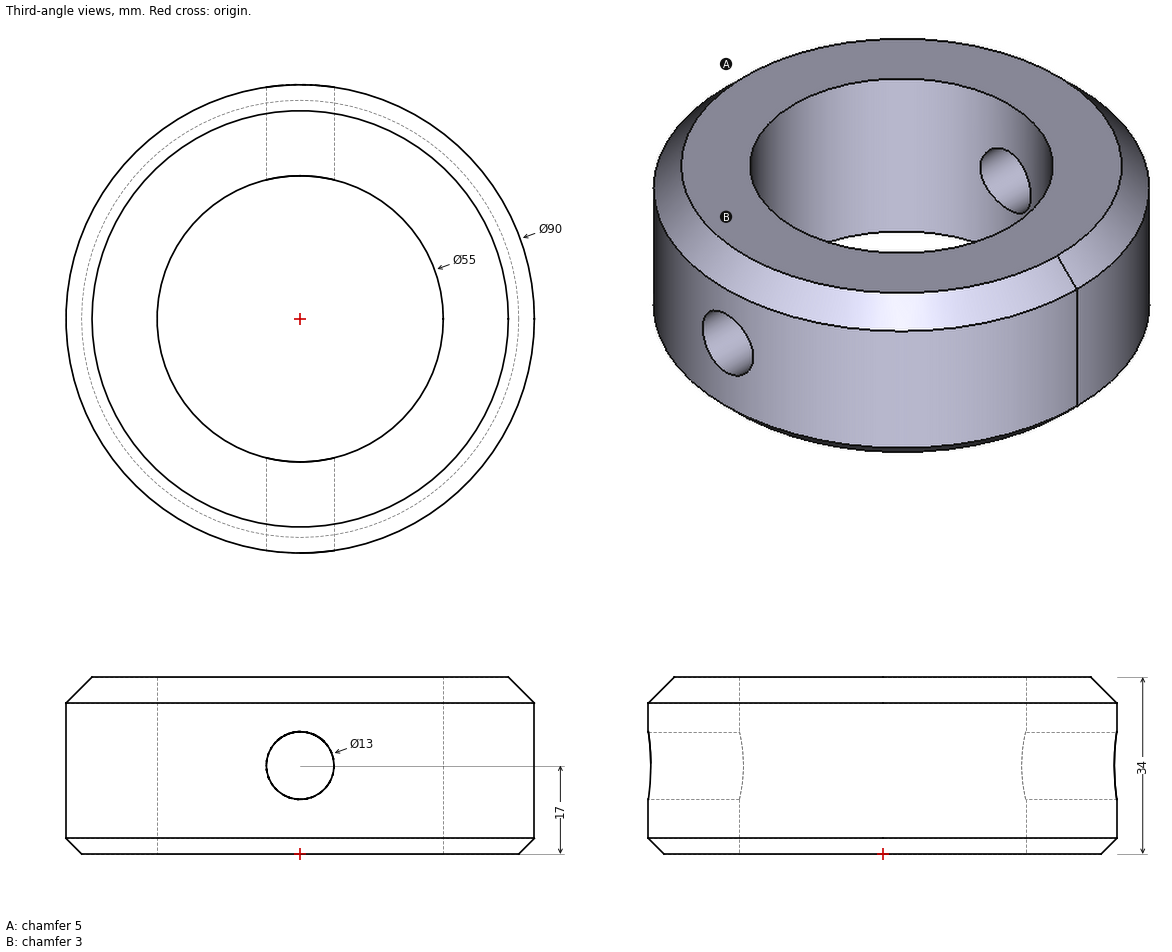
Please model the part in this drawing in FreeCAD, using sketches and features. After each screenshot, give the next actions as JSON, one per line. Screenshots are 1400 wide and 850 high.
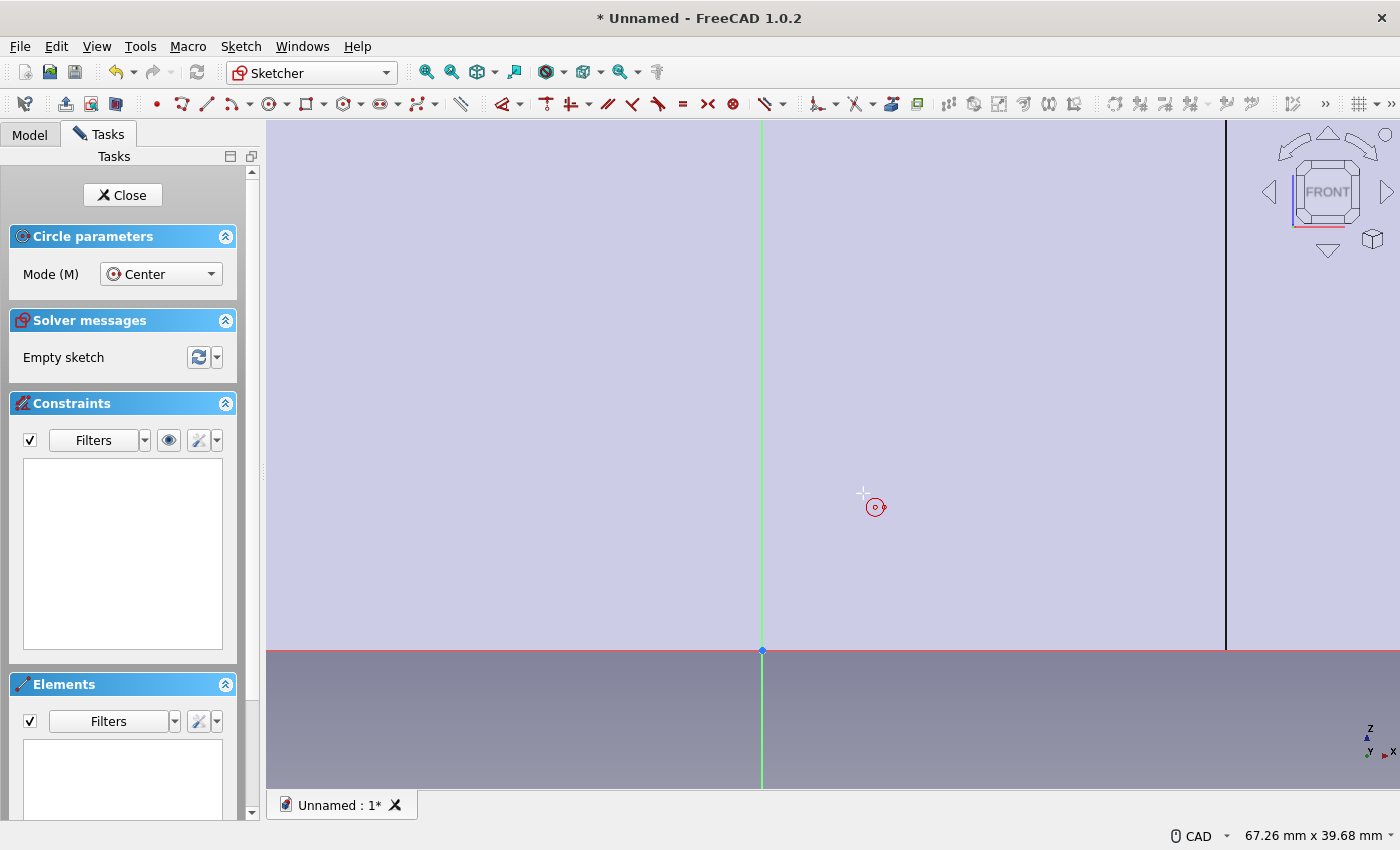
{"action": "left_click", "coordinate": [762, 364]}
{"action": "left_click", "coordinate": [840, 286]}
{"action": "key", "text": "Escape"}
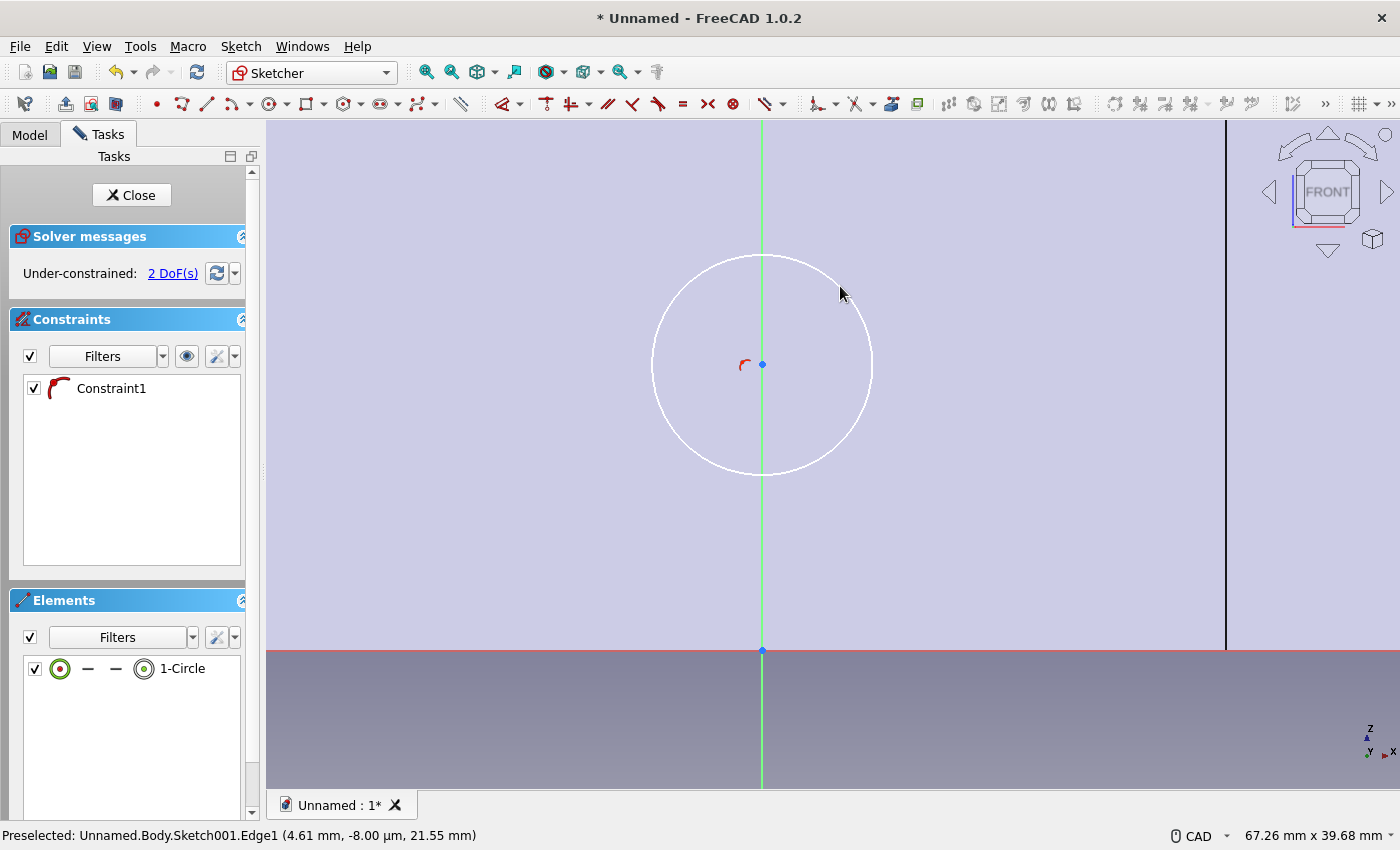
{"action": "key", "text": "d"}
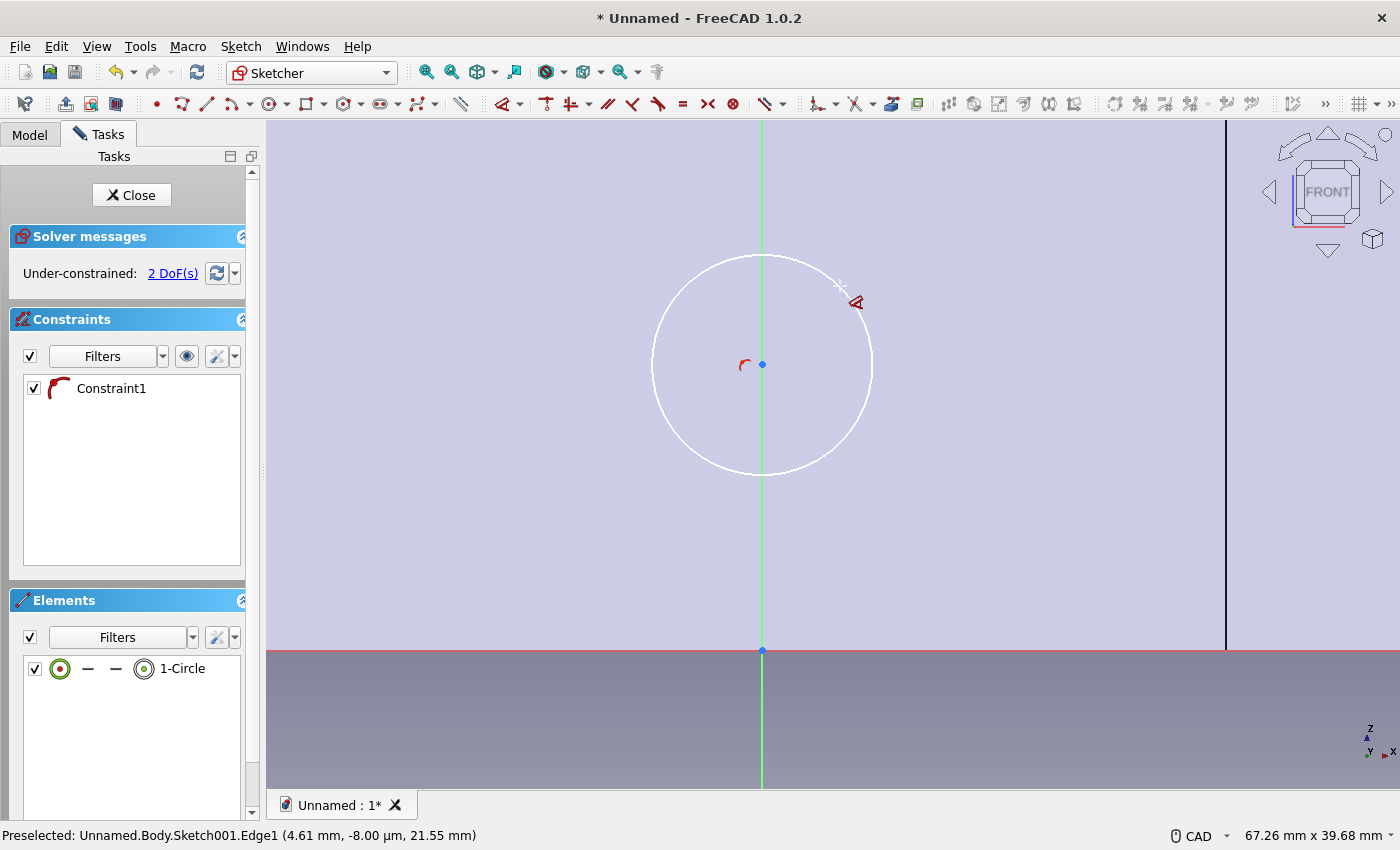
{"action": "left_click", "coordinate": [840, 287]}
{"action": "left_click", "coordinate": [863, 264]}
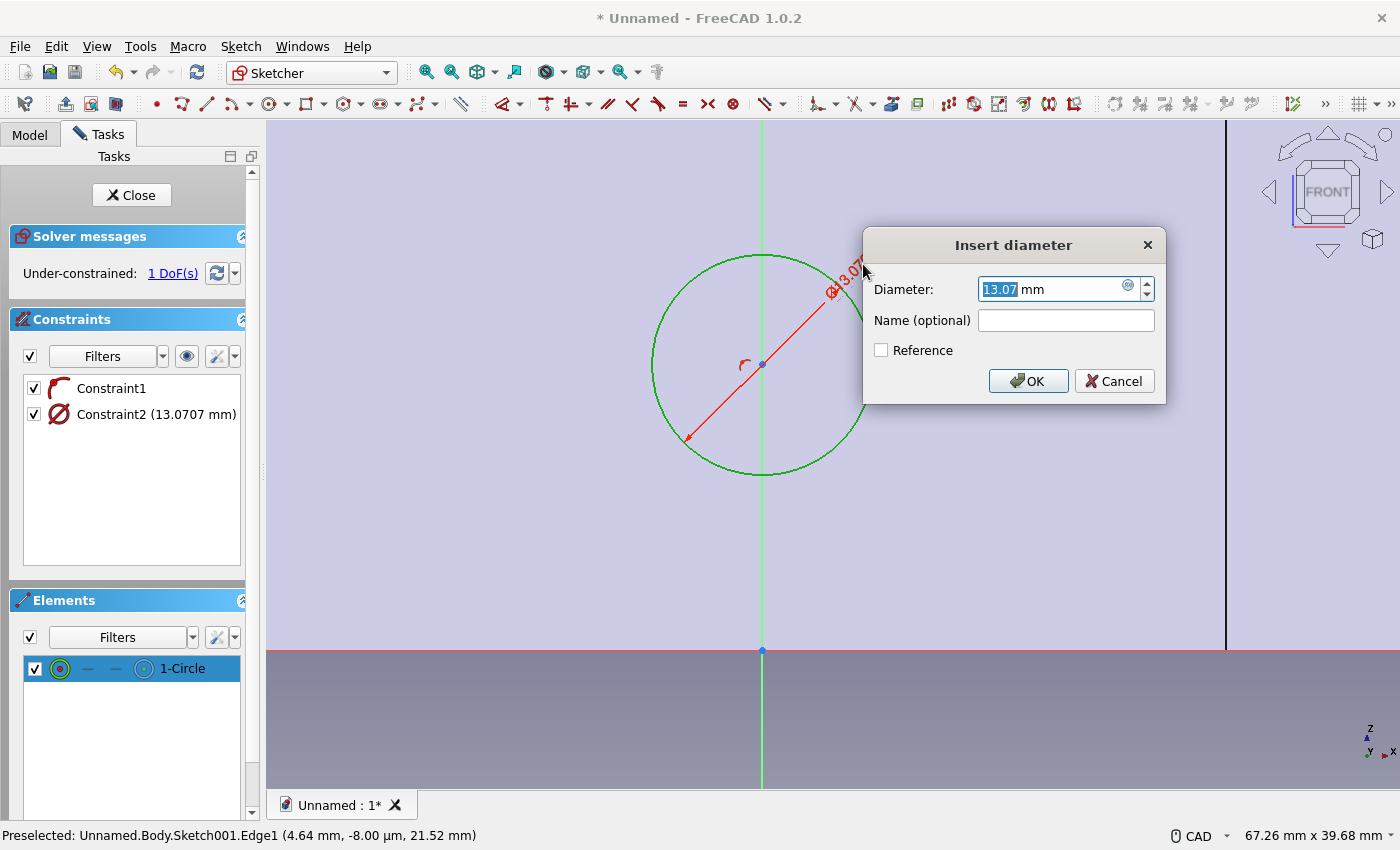
{"action": "type", "text": "13"}
{"action": "key", "text": "Return"}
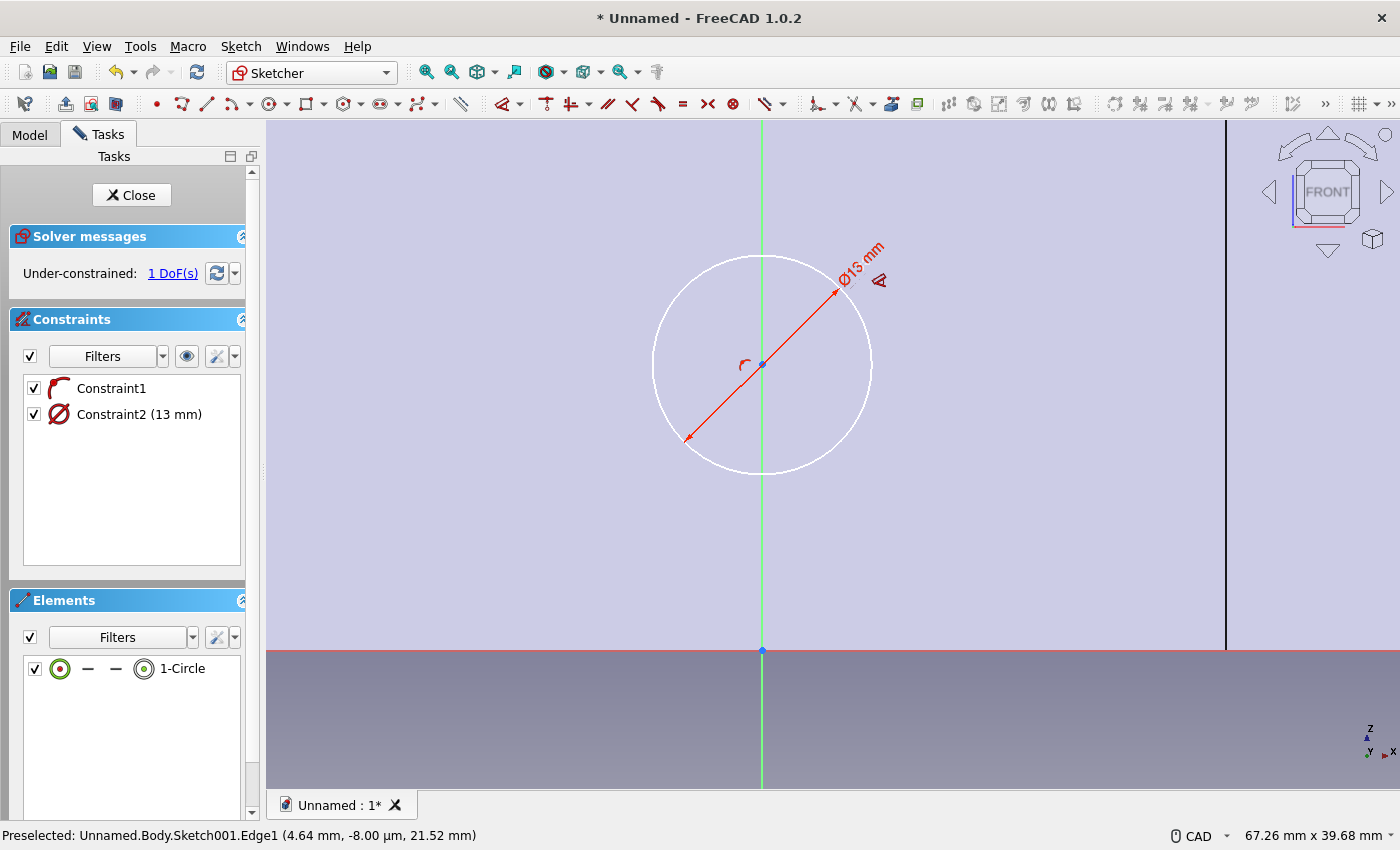
{"action": "left_click", "coordinate": [762, 365]}
{"action": "left_click", "coordinate": [796, 508]}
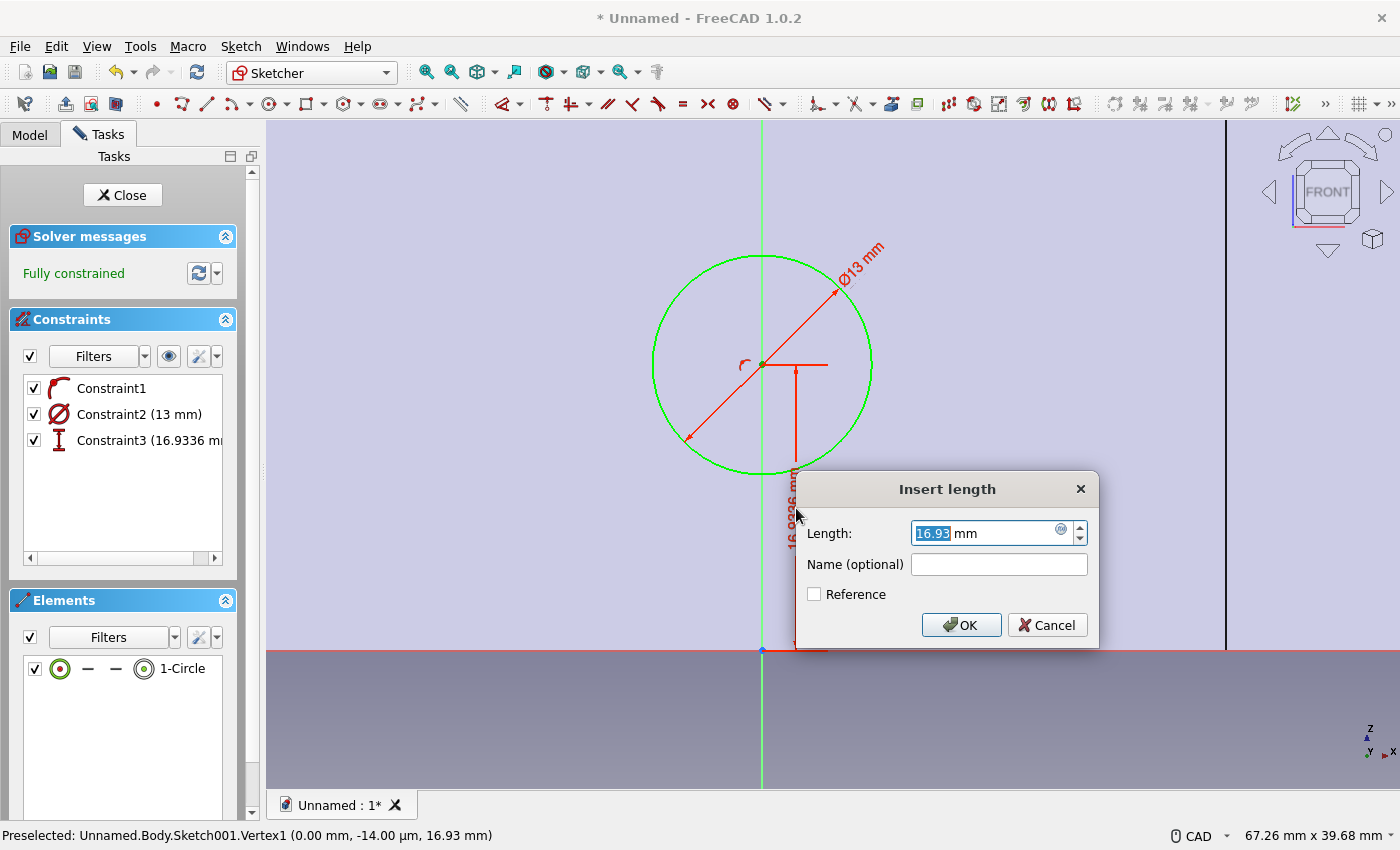
{"action": "type", "text": "17"}
{"action": "key", "text": "Return"}
{"action": "key", "text": "Escape"}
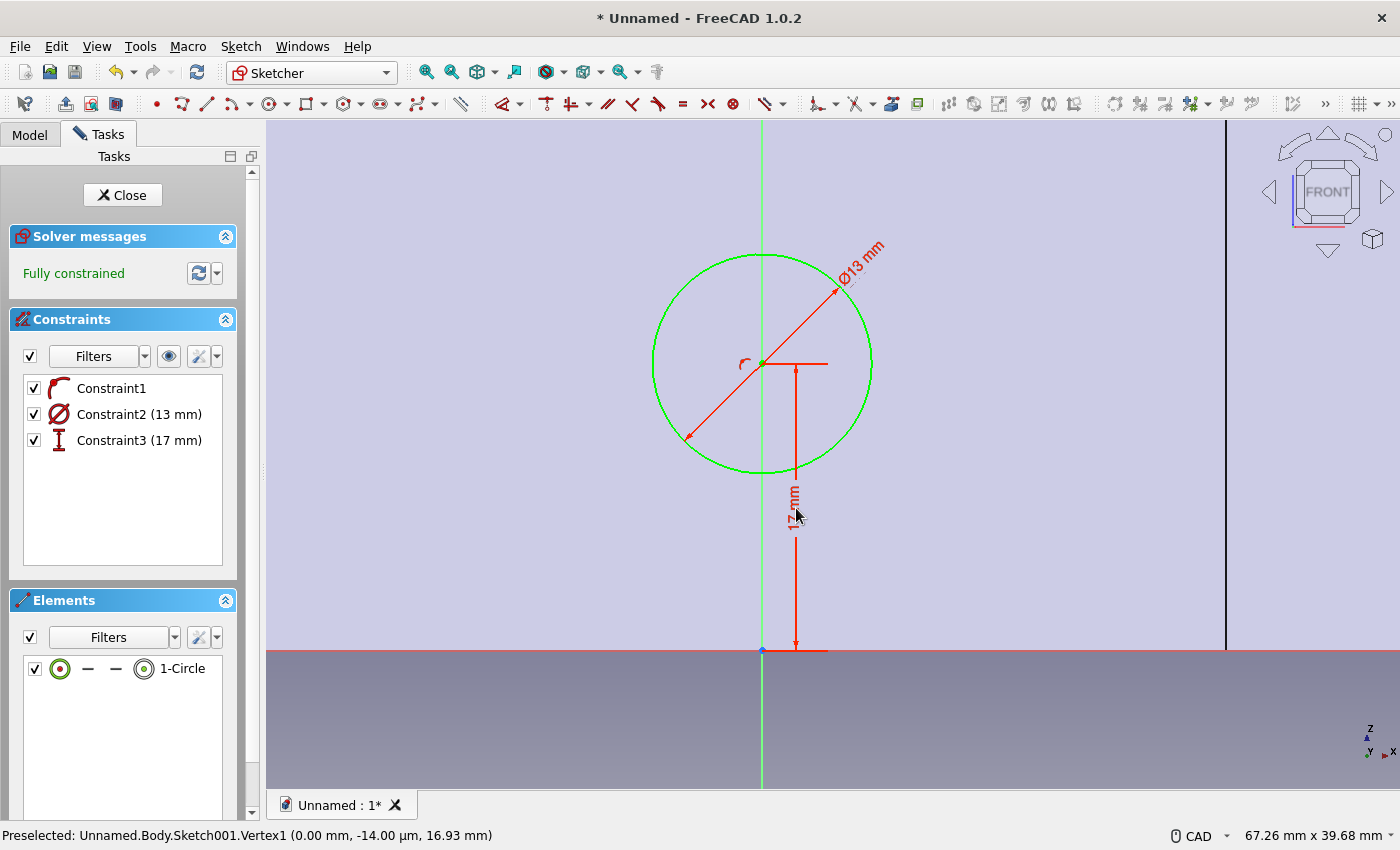
{"action": "left_click", "coordinate": [123, 195]}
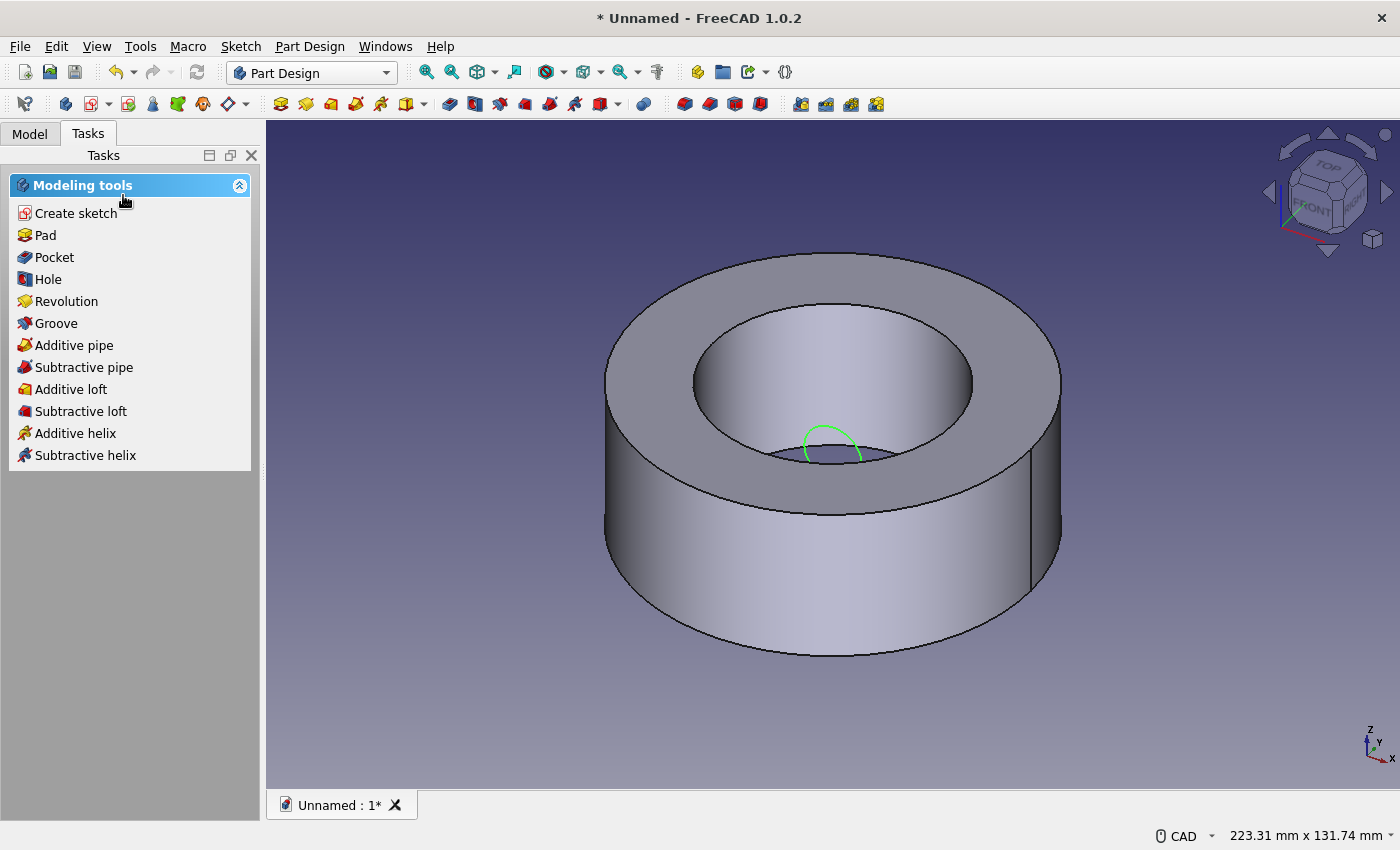
{"action": "left_click", "coordinate": [450, 104]}